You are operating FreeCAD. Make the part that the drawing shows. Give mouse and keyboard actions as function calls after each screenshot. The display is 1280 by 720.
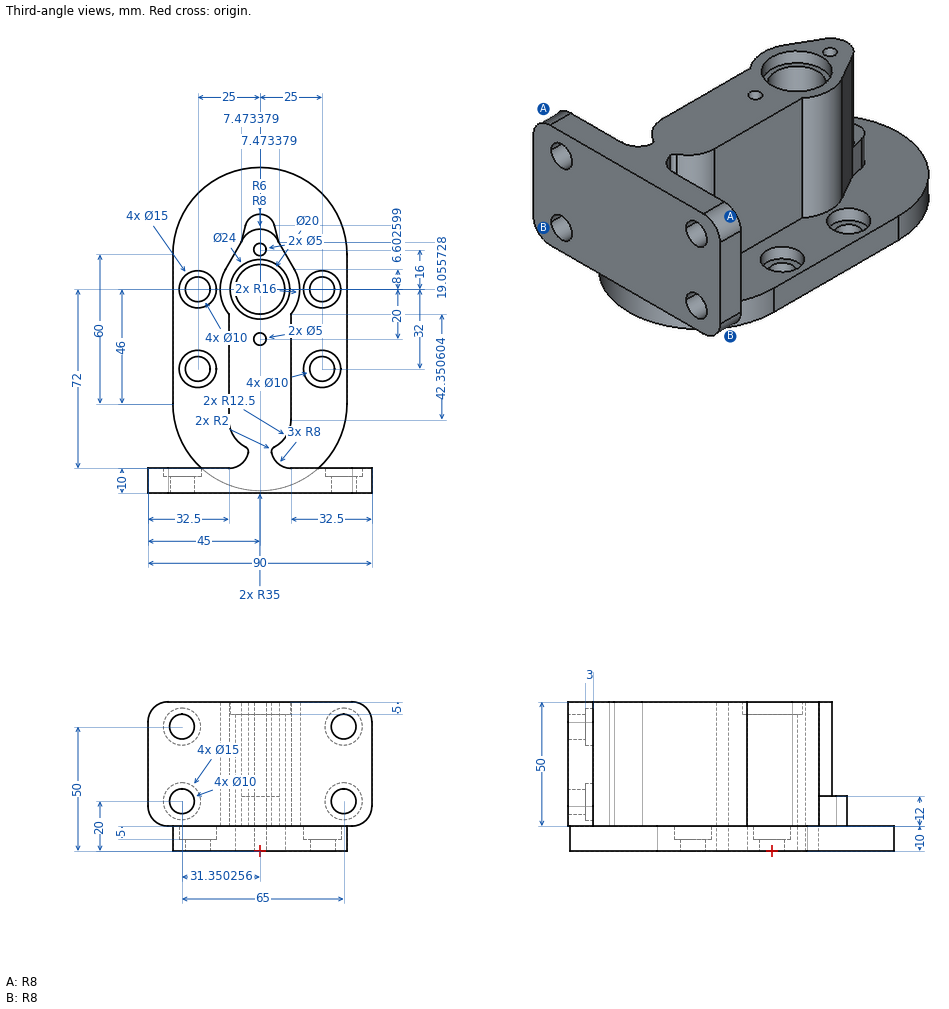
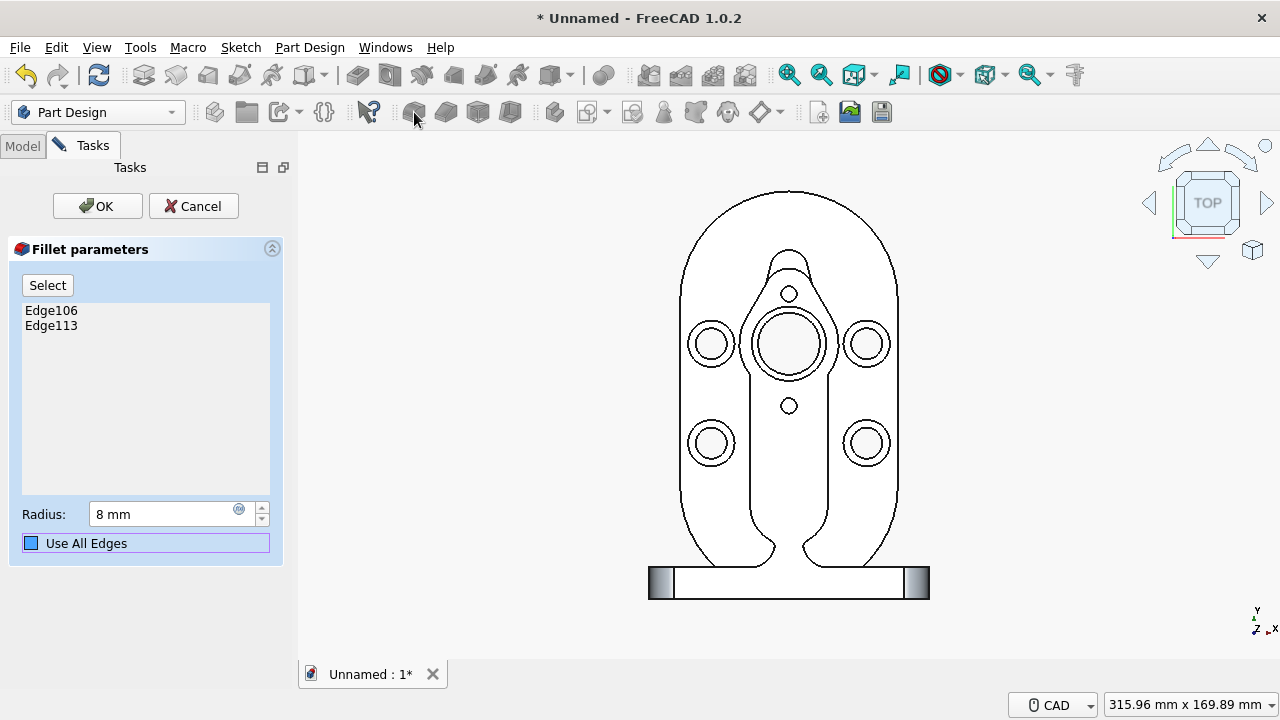
click(98, 206)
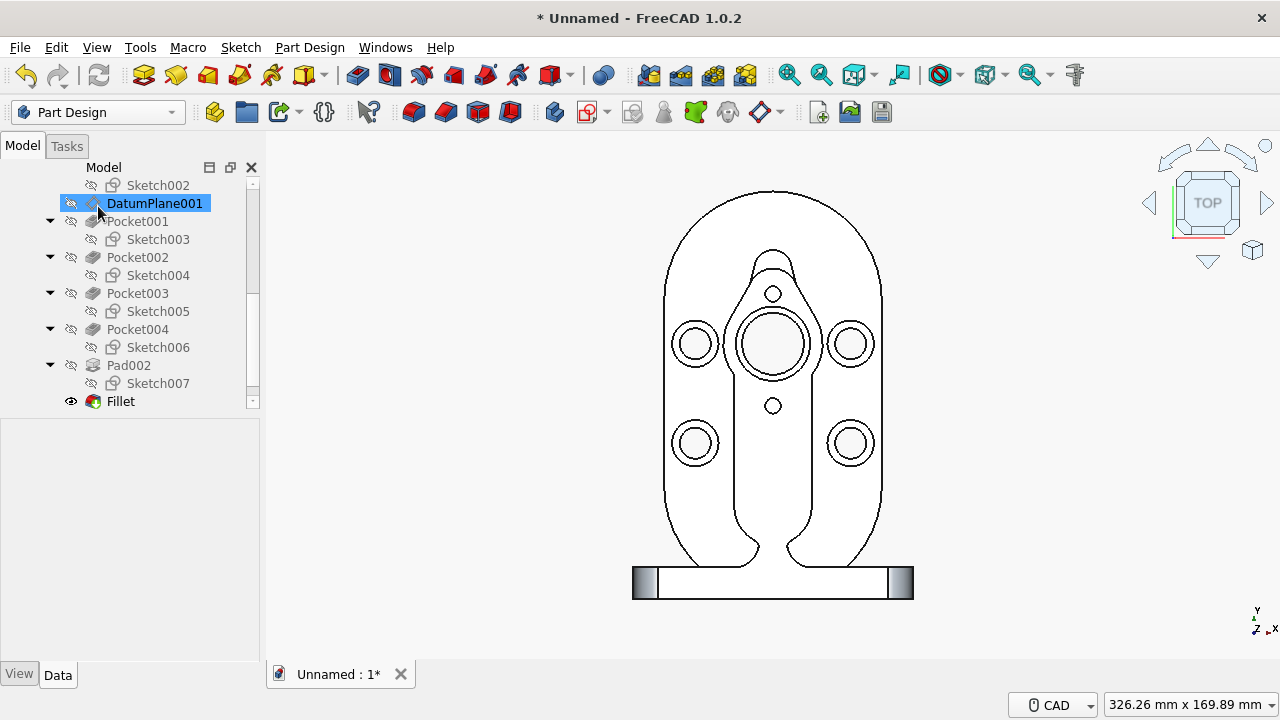
key(0)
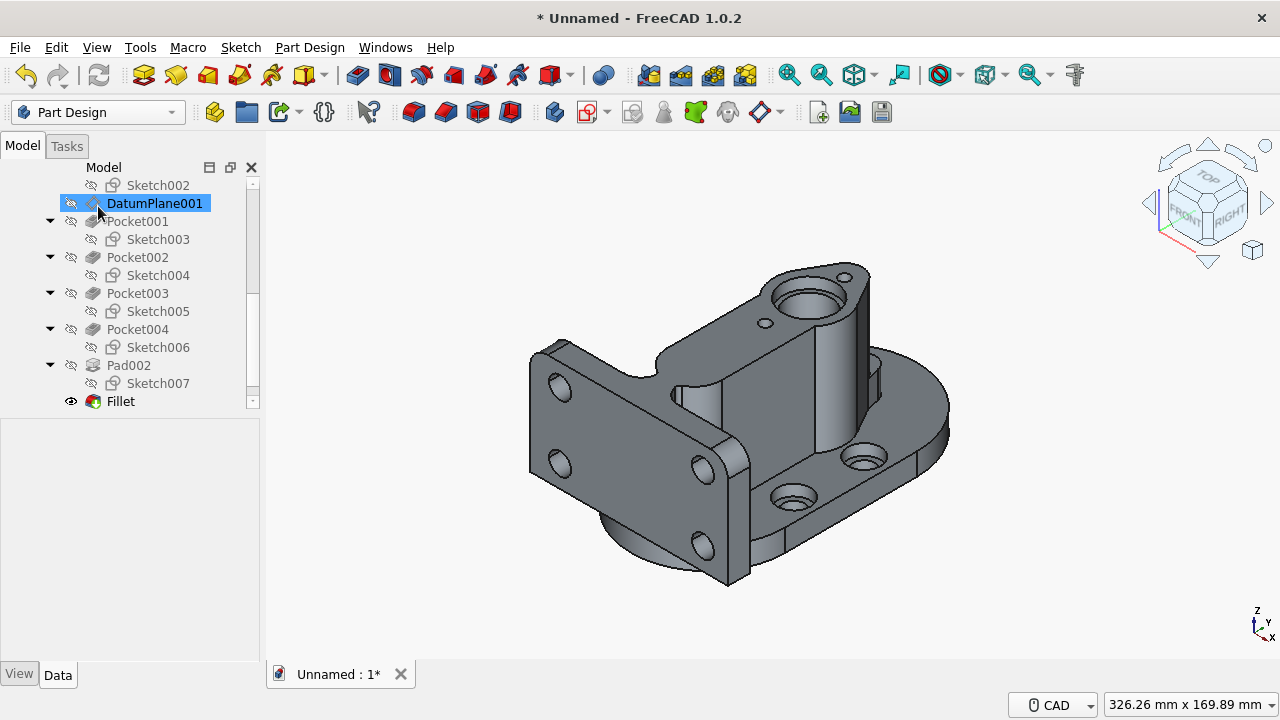
key(2)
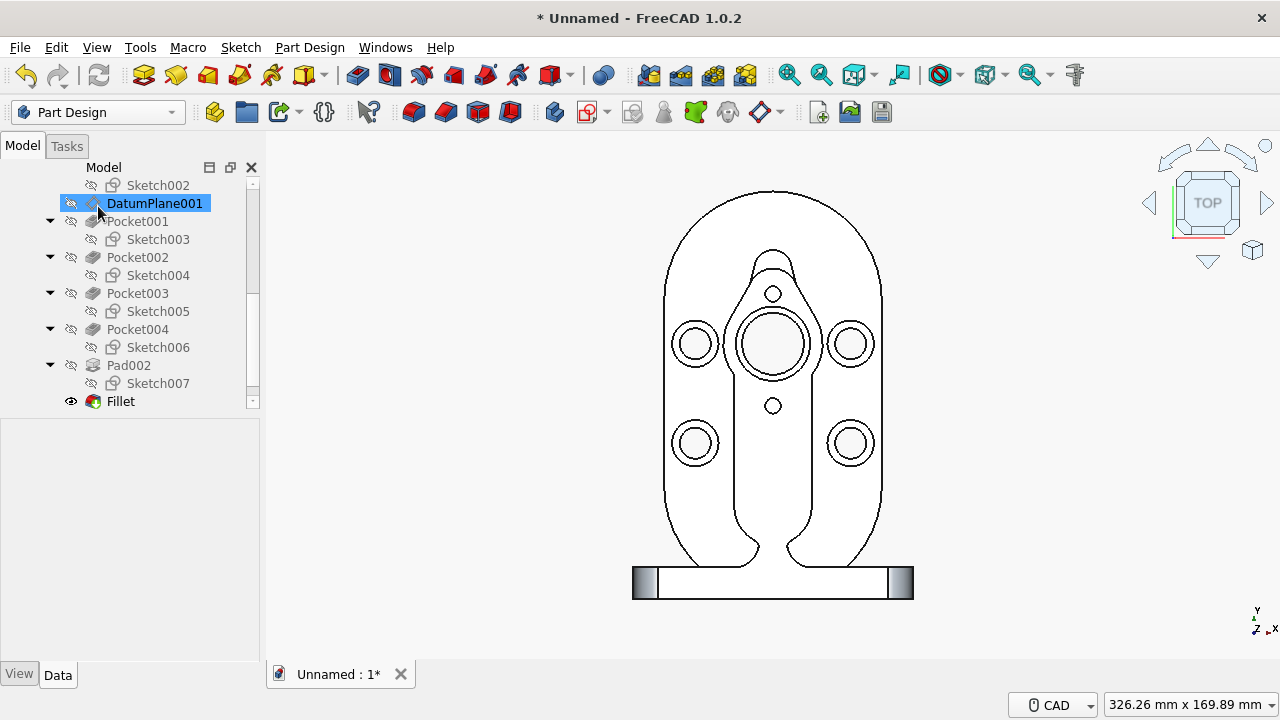
key(1)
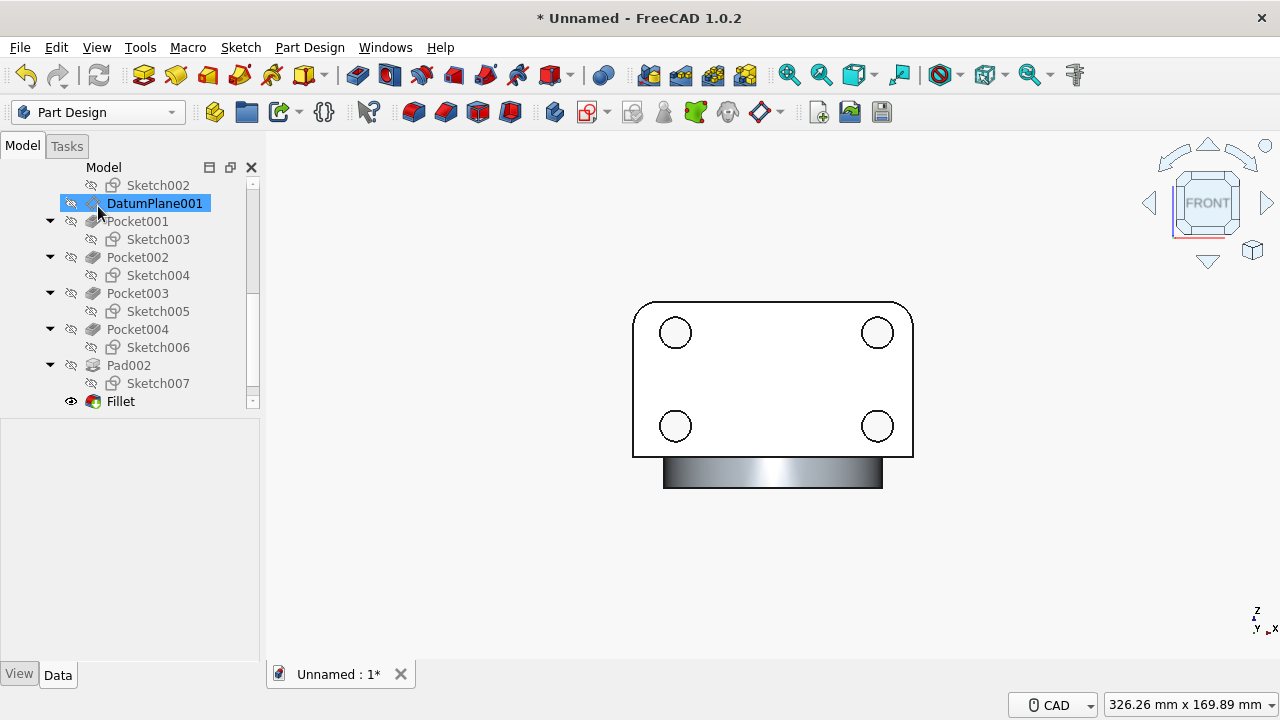
click(790, 76)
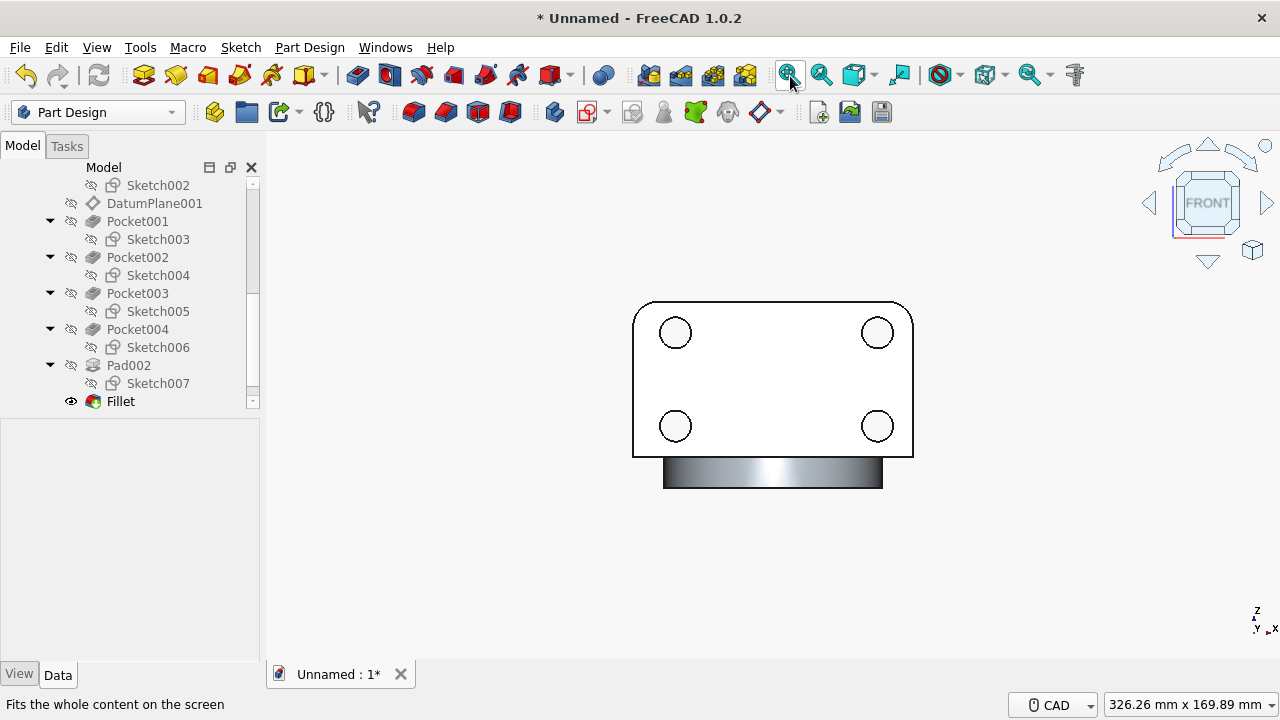
key(3)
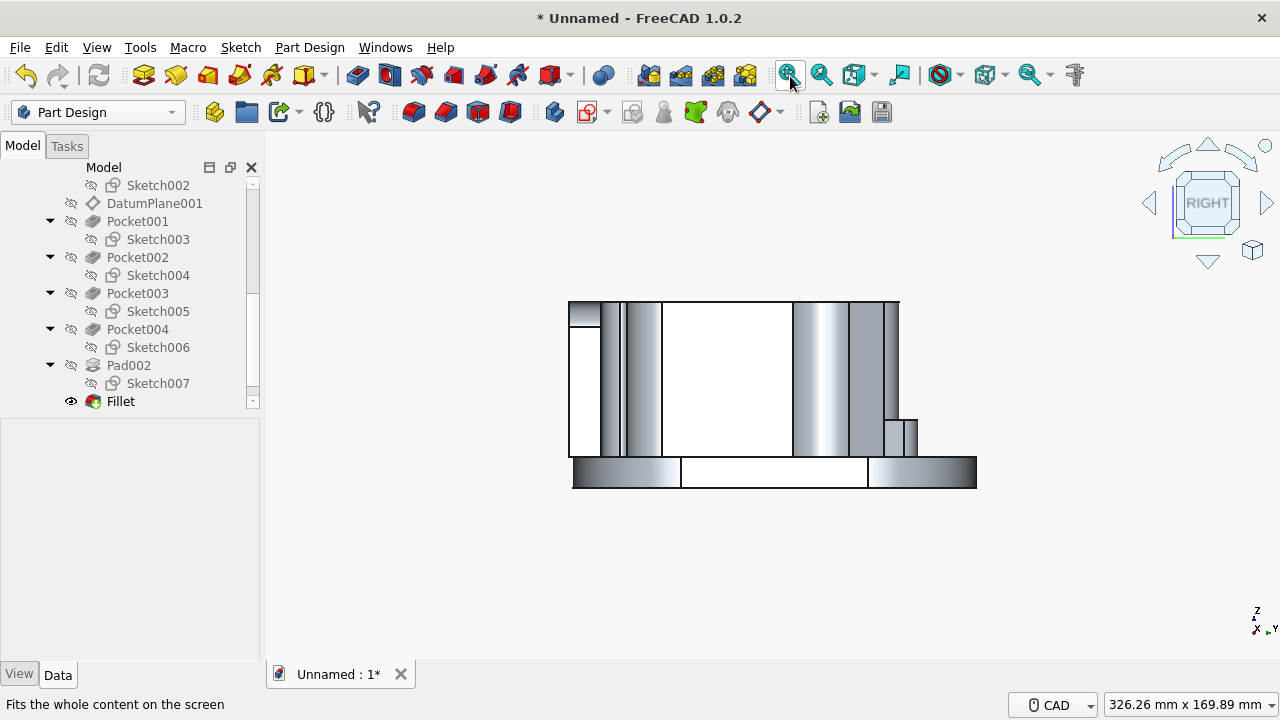
click(790, 76)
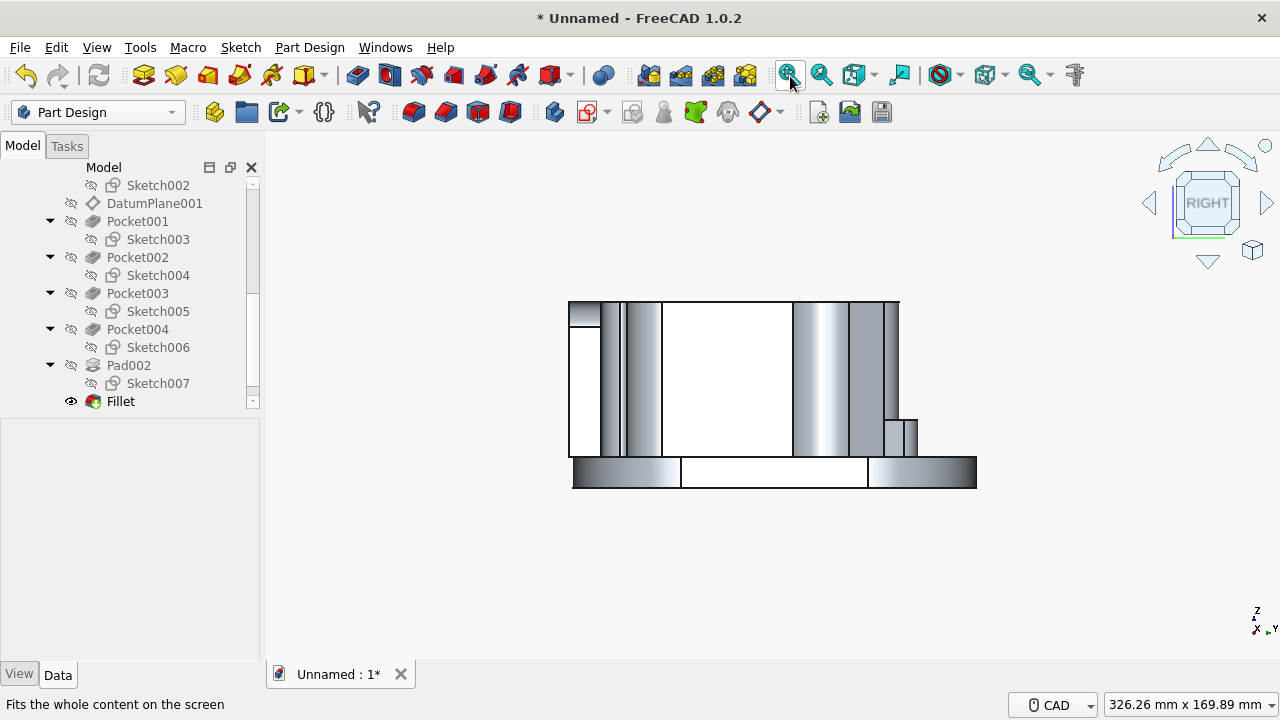
click(585, 456)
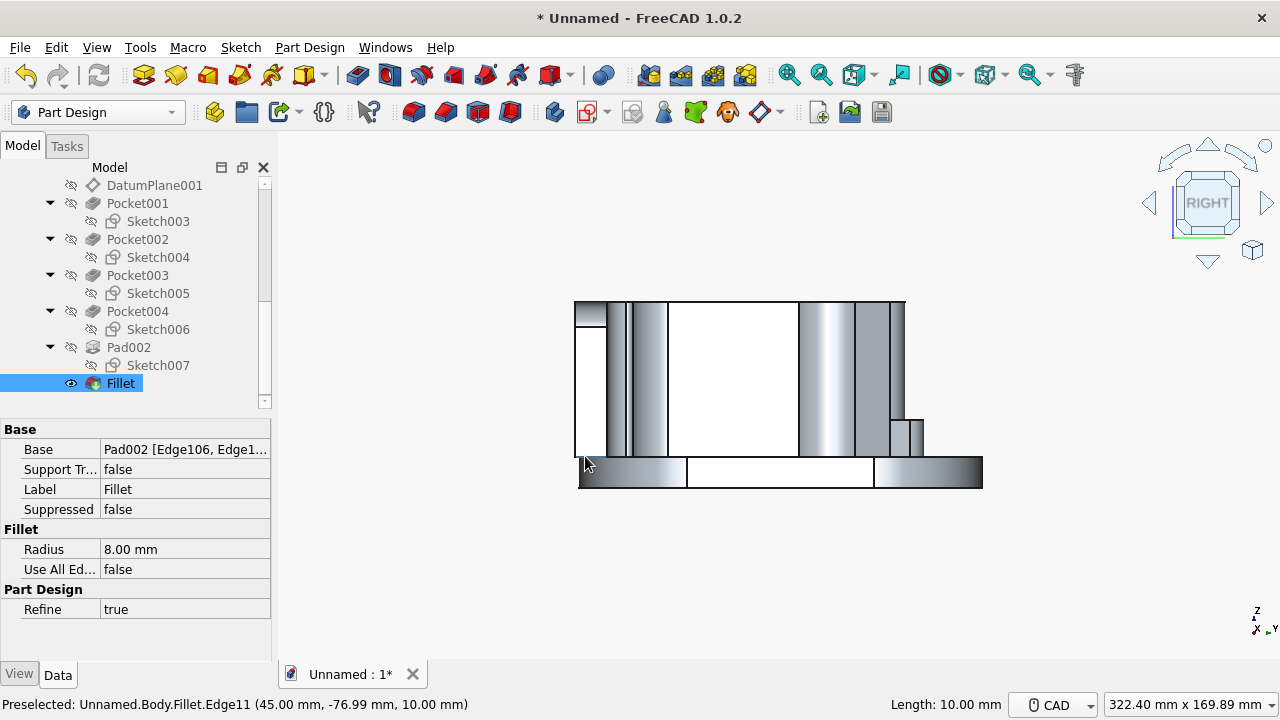
key(5)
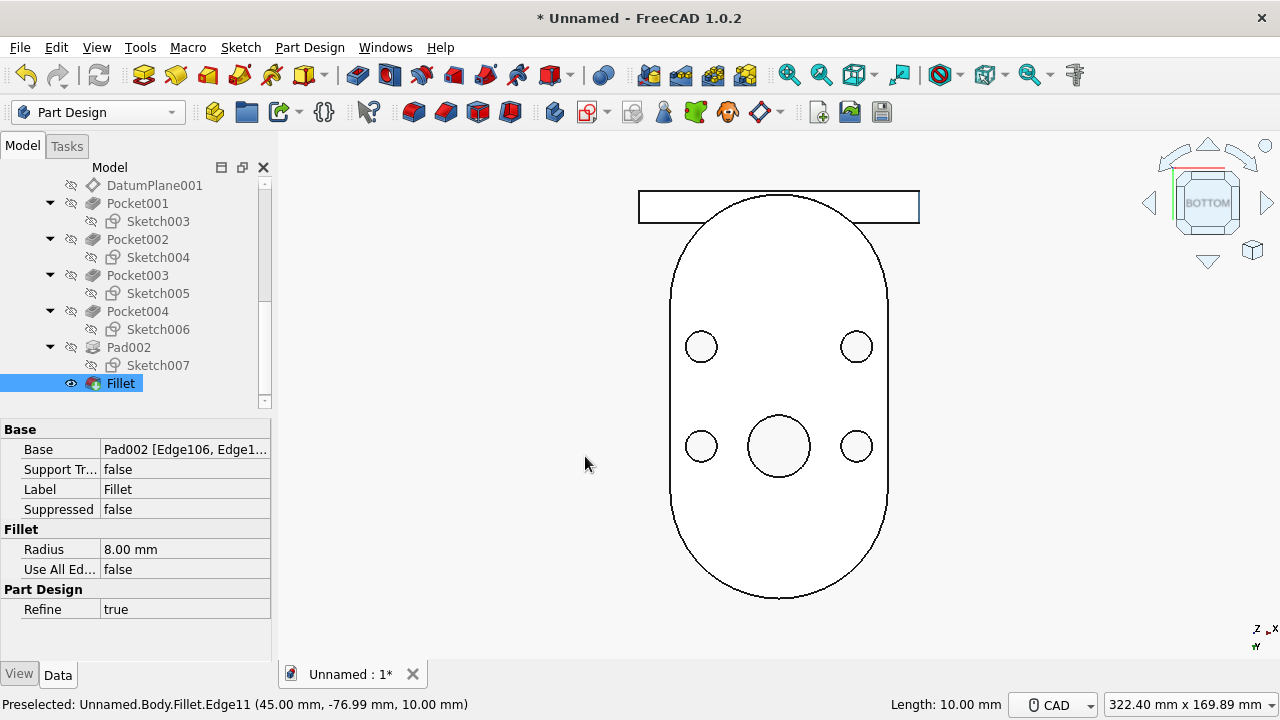
click(639, 206, ctrl)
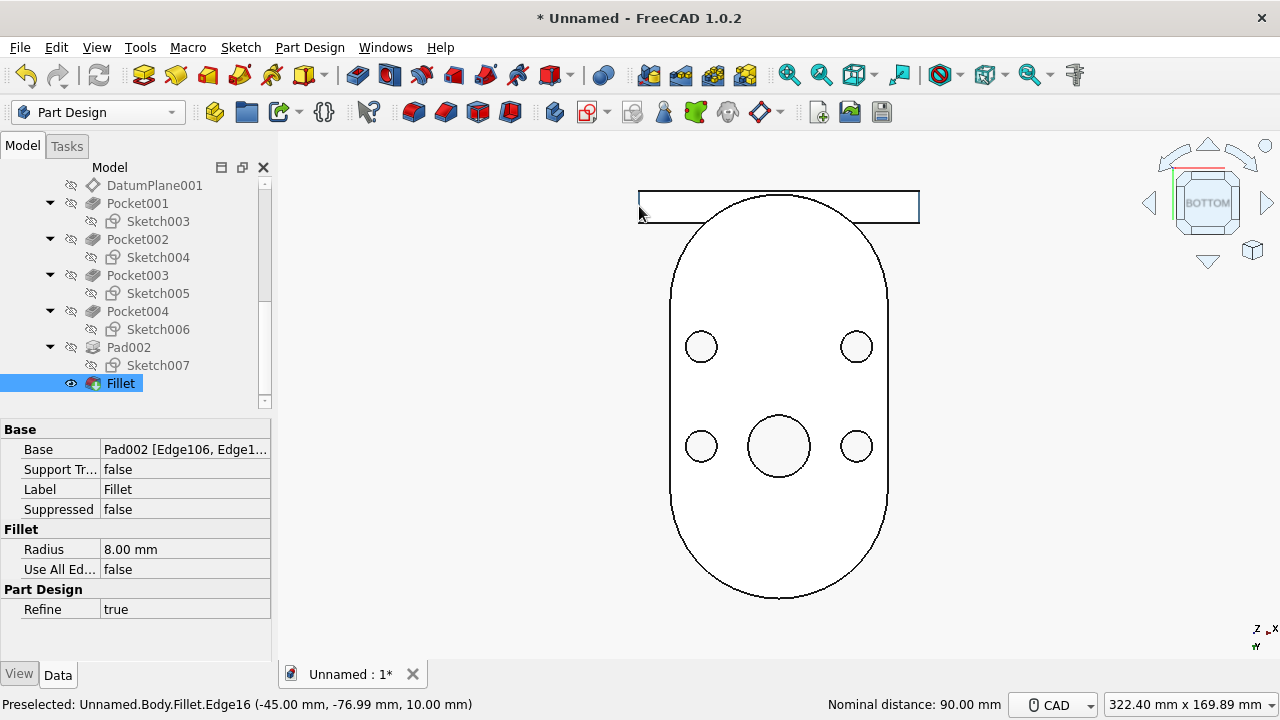
click(414, 112)